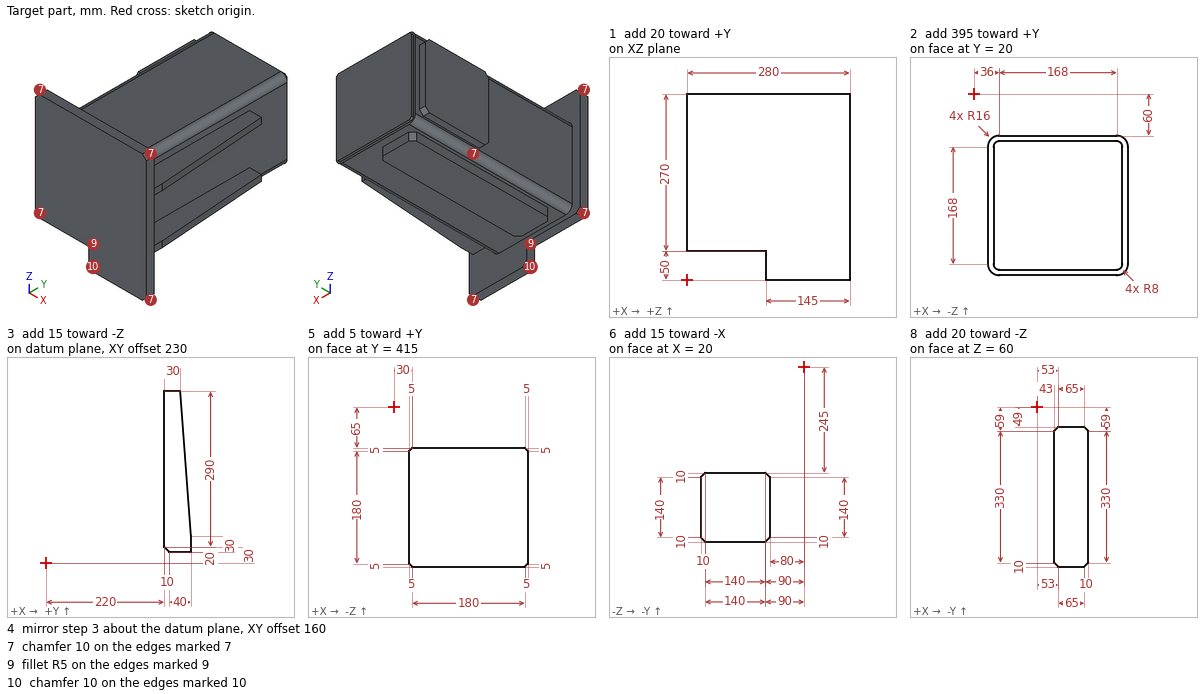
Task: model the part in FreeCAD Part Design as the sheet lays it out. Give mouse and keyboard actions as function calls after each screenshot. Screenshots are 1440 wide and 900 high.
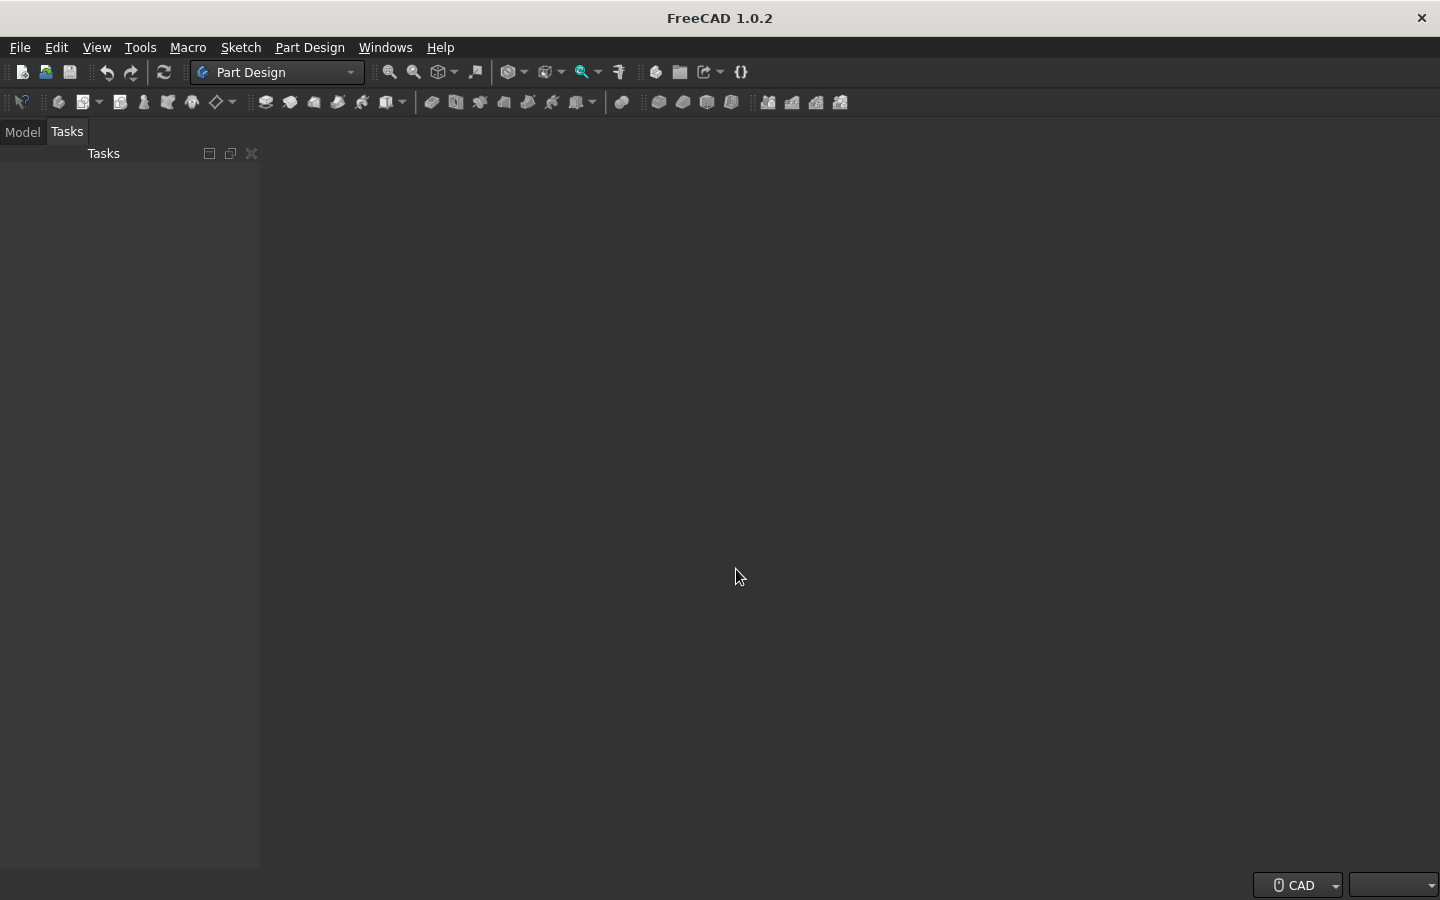
key(ctrl+n)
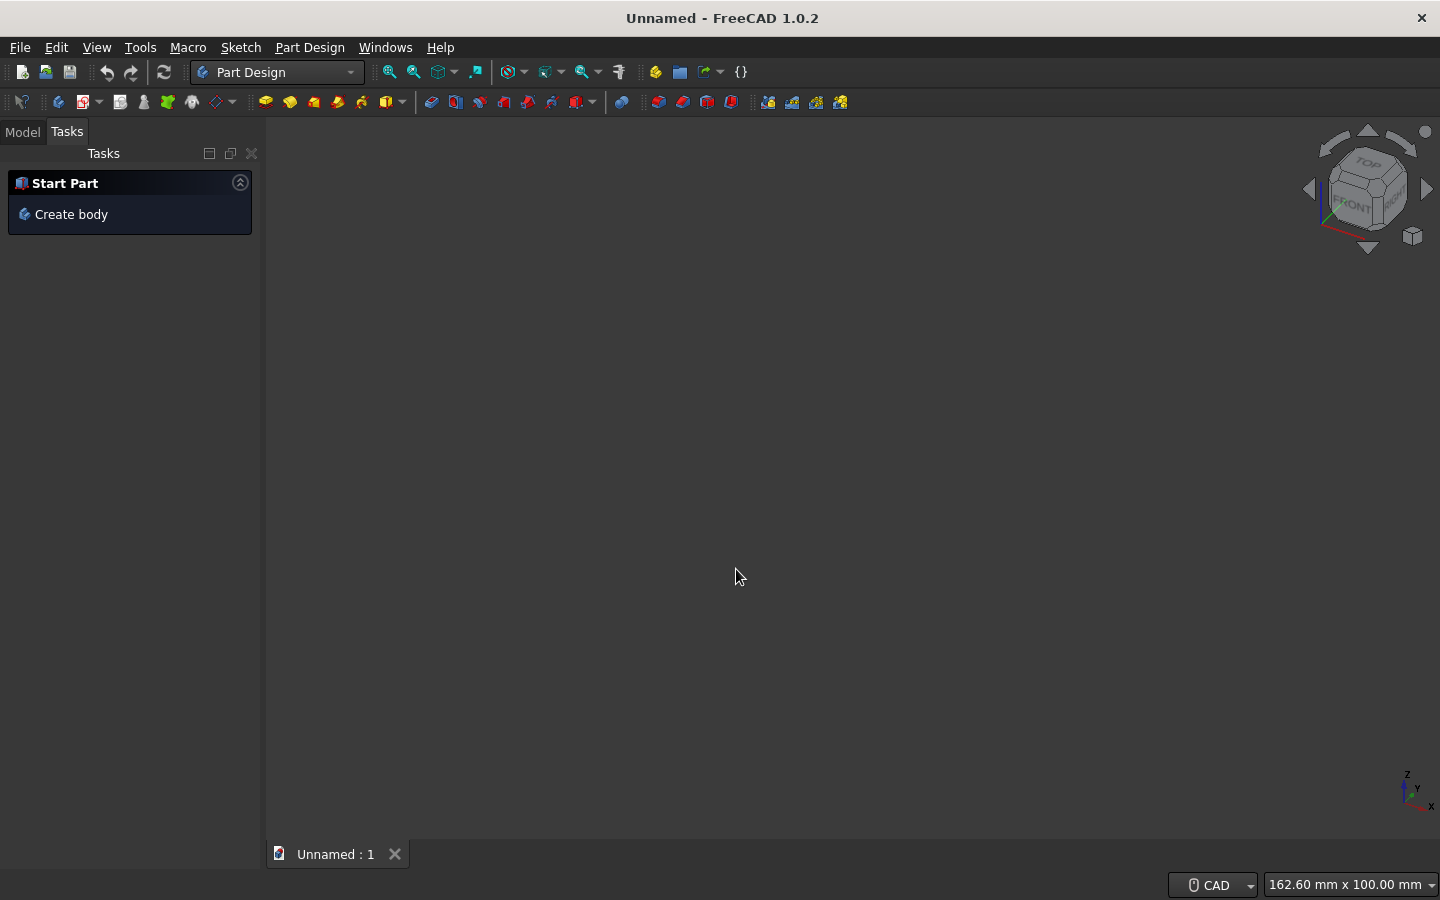
click(84, 102)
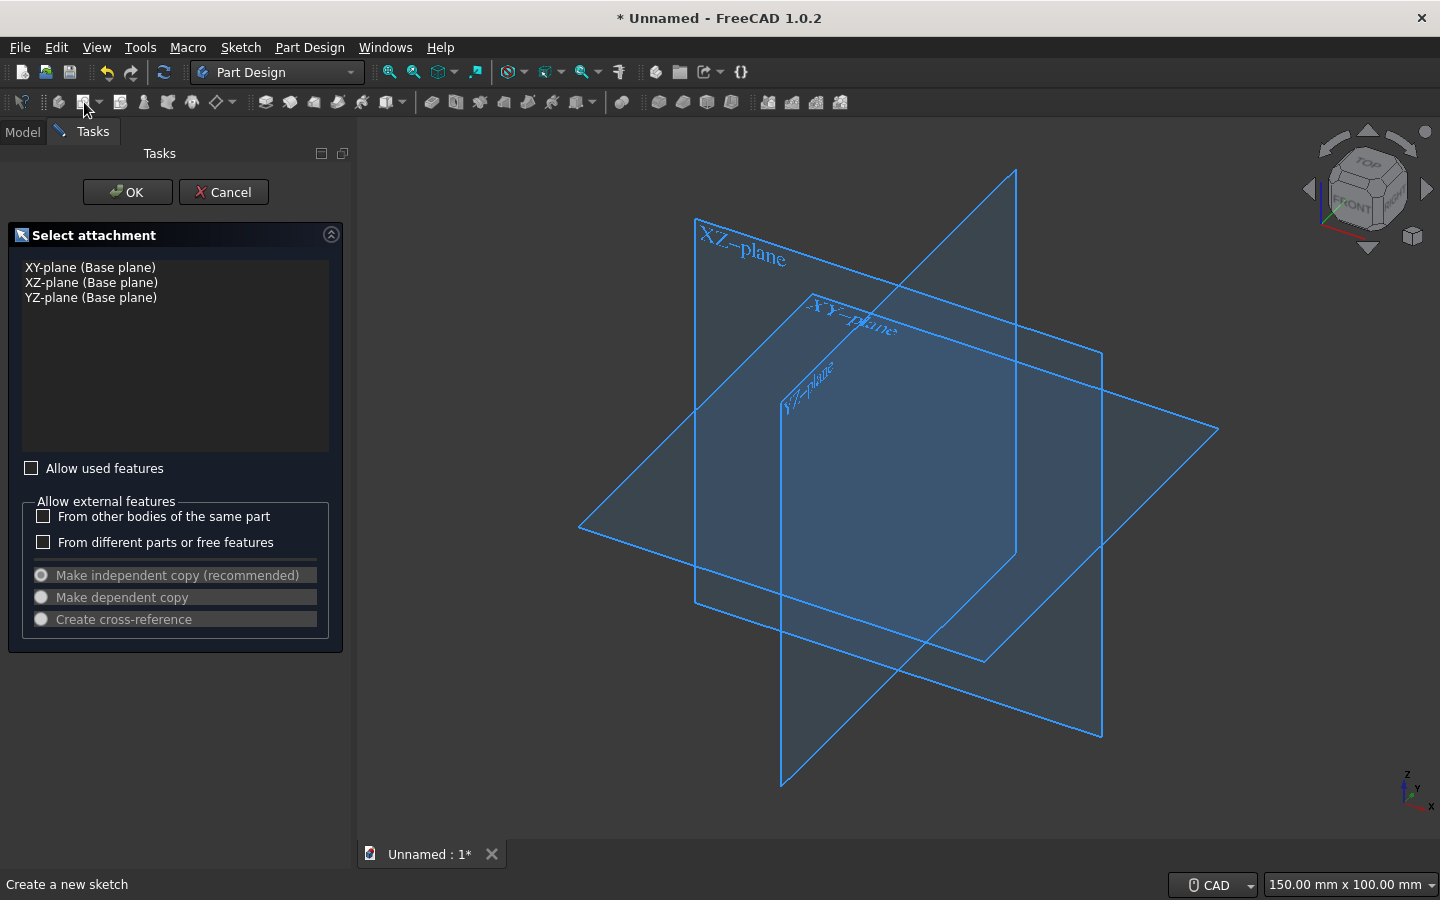
click(82, 282)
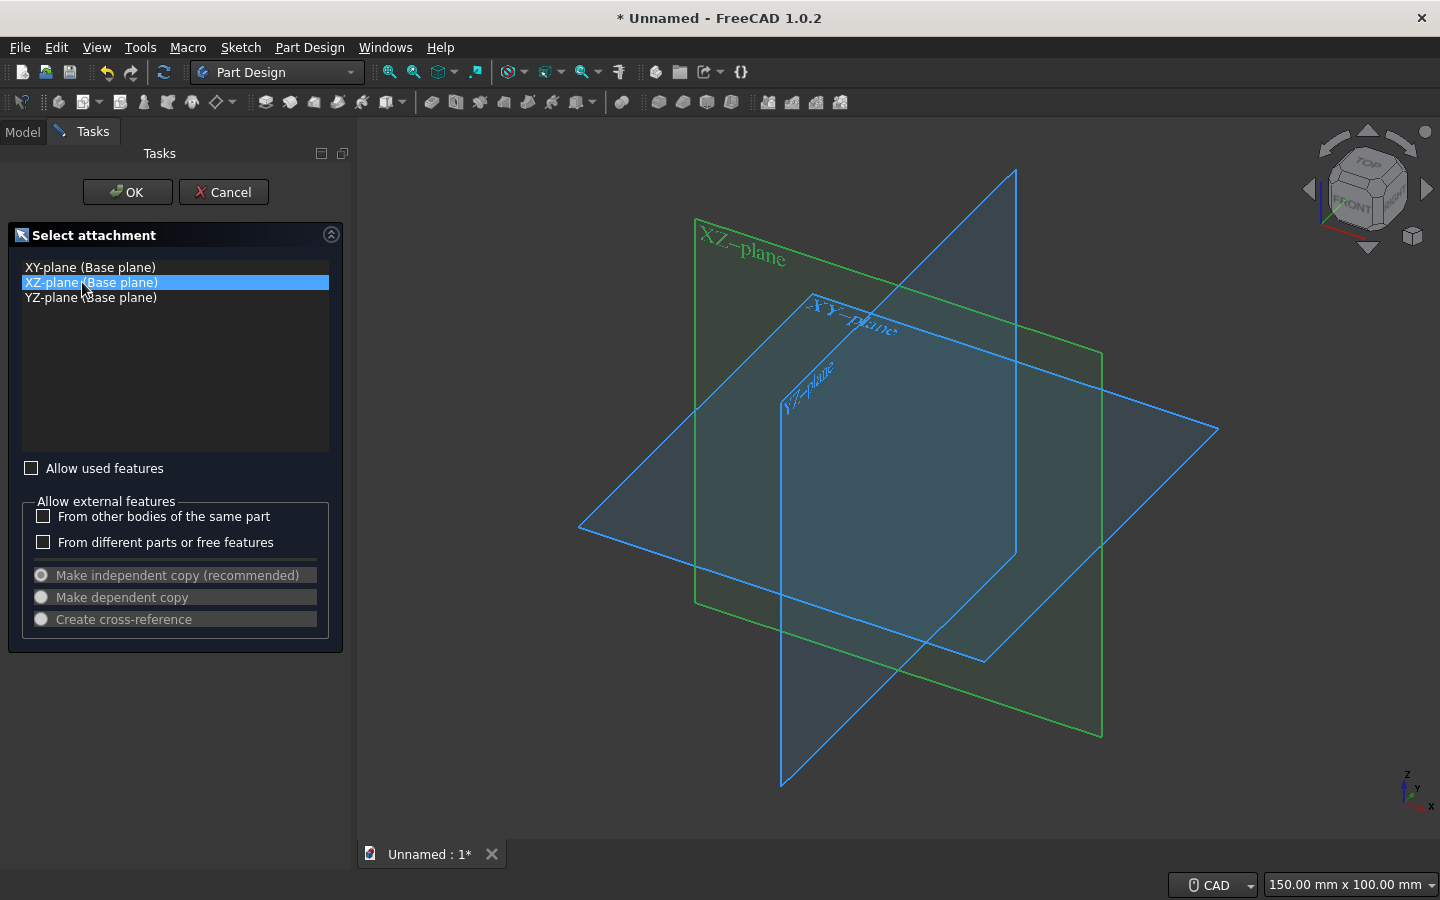
click(128, 192)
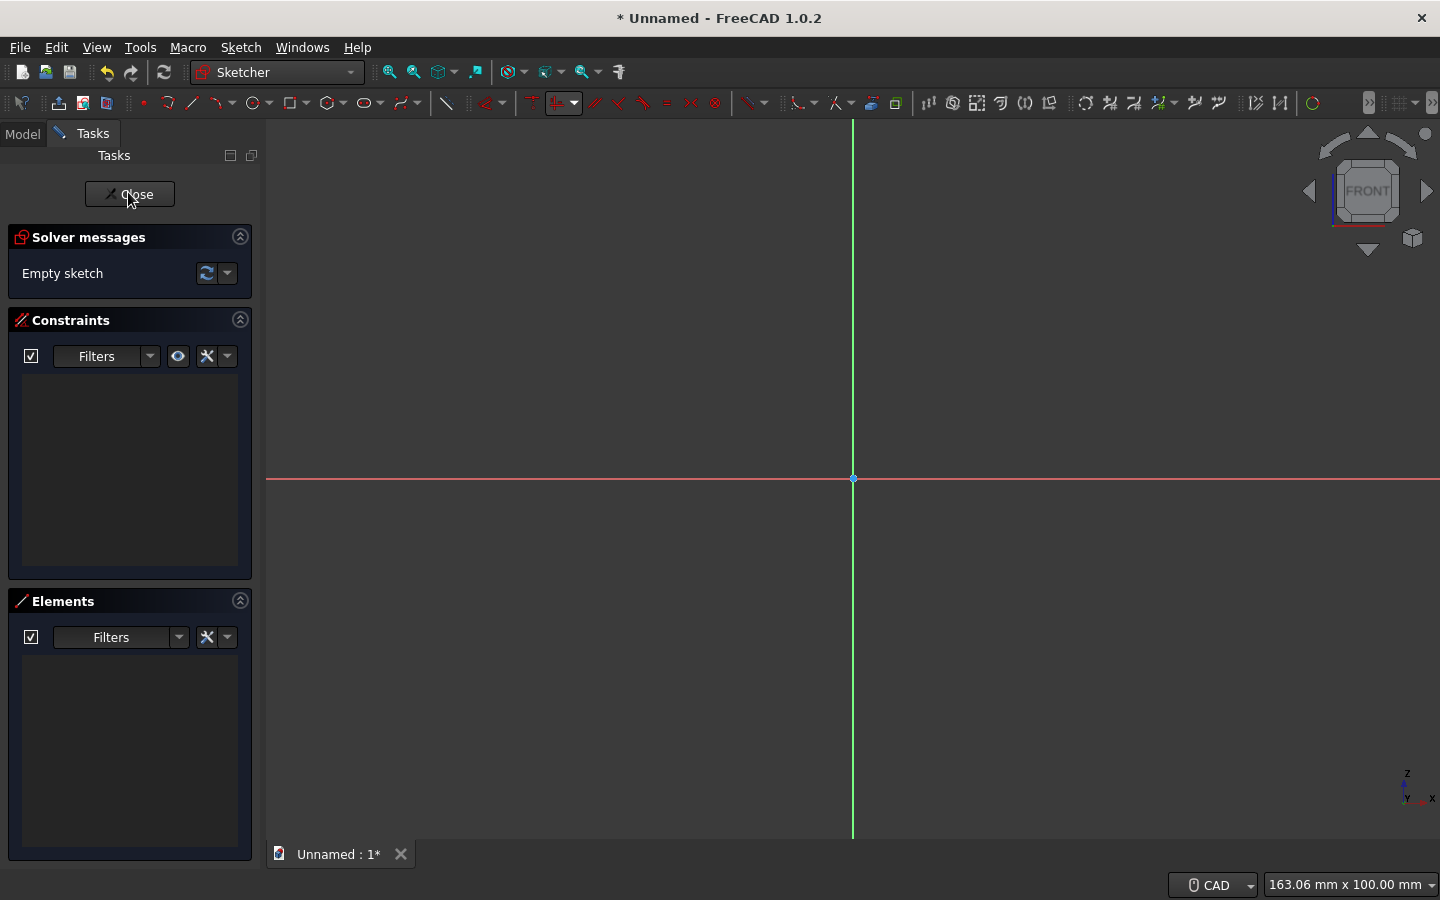
scroll(512, 770, down, 8)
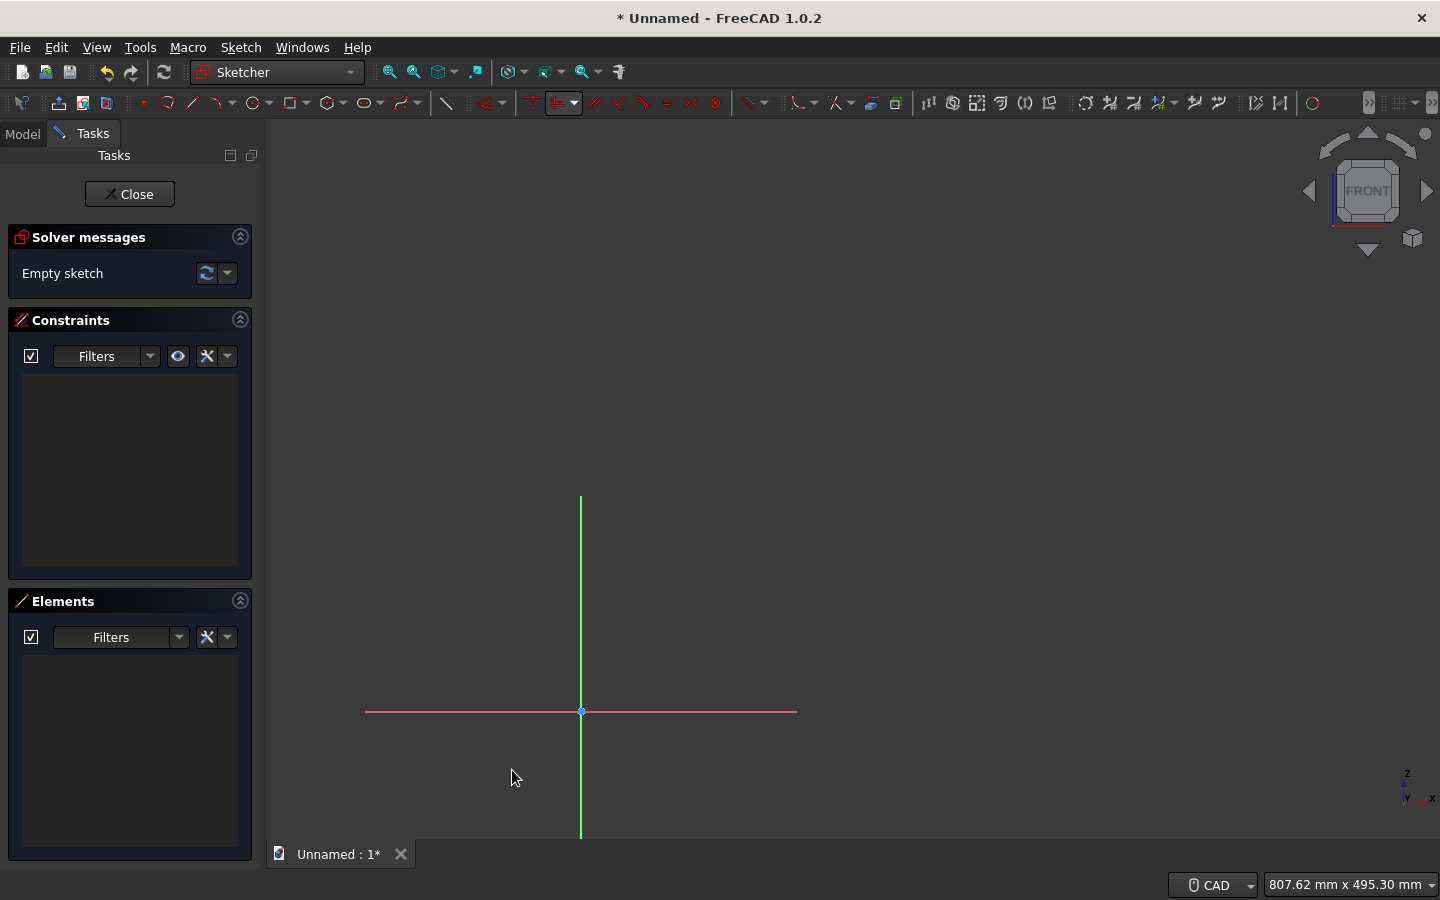
click(168, 104)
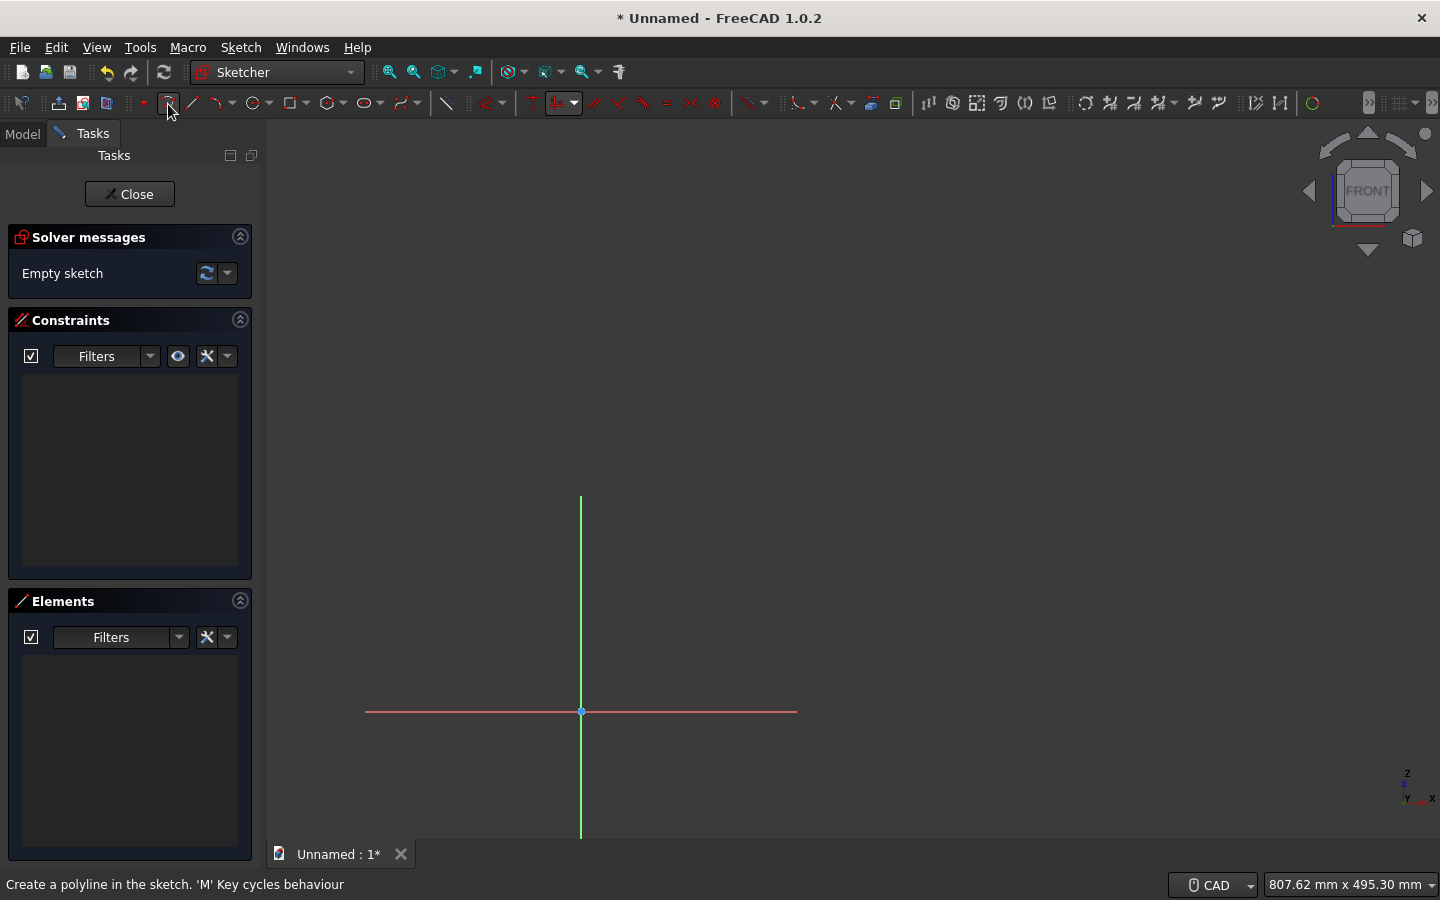
click(581, 639)
click(590, 247)
click(988, 247)
click(988, 712)
click(777, 703)
click(777, 639)
click(581, 640)
key(Escape)
key(Escape)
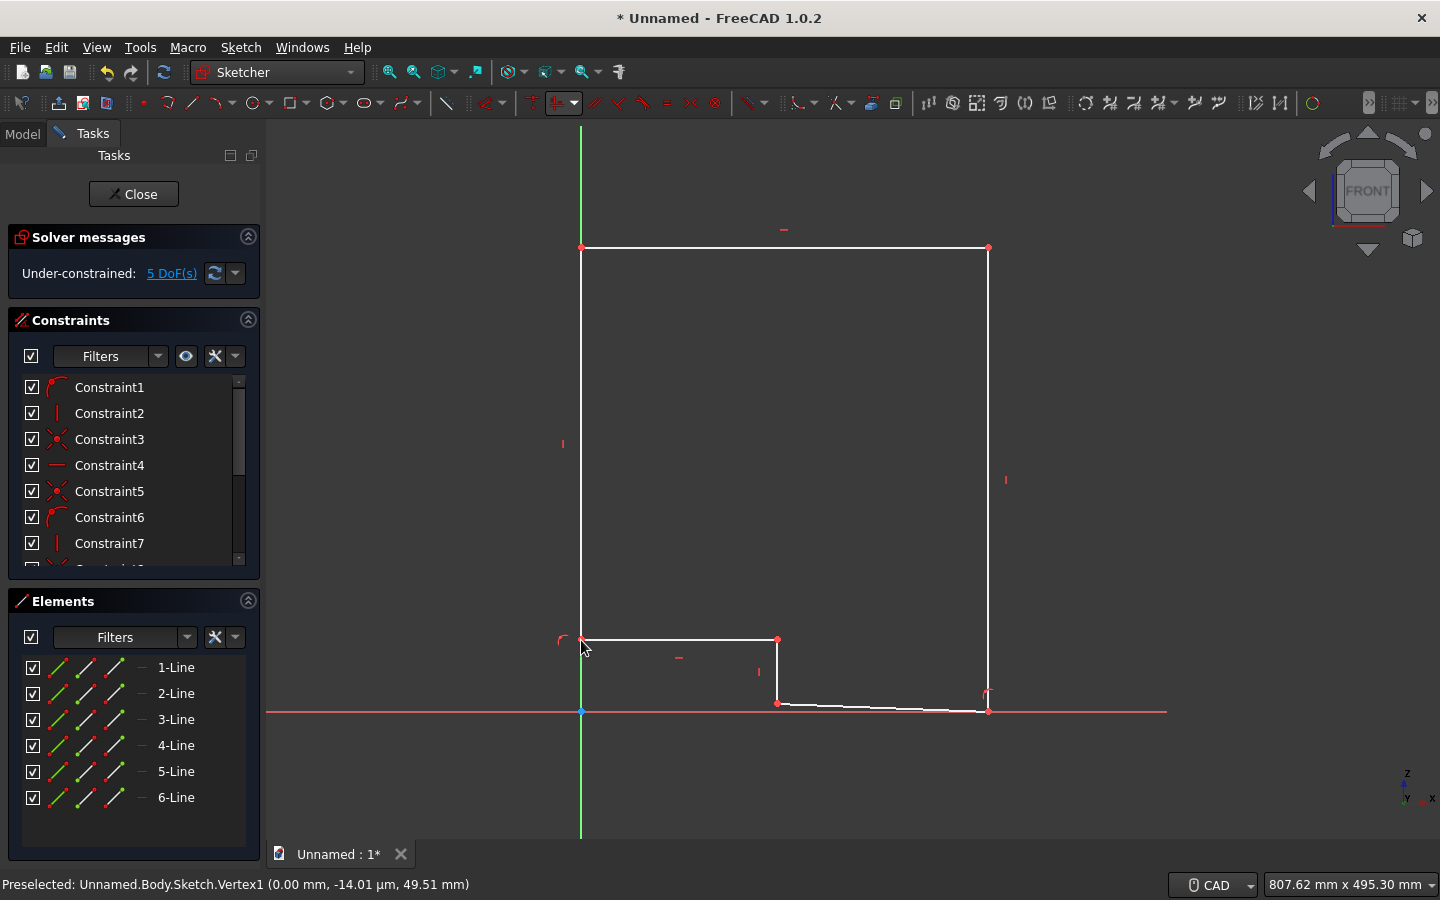
click(925, 710)